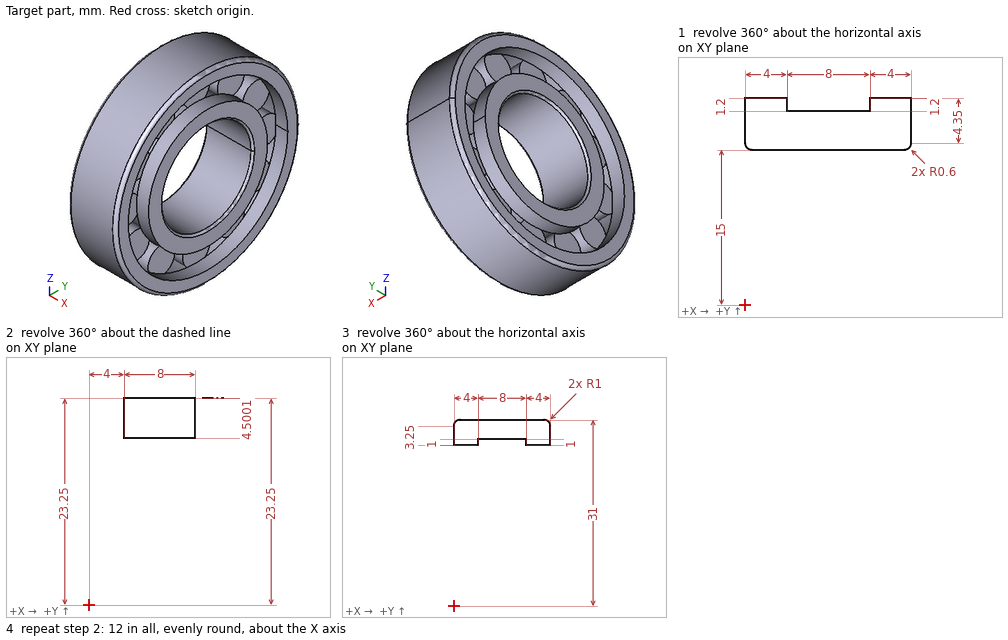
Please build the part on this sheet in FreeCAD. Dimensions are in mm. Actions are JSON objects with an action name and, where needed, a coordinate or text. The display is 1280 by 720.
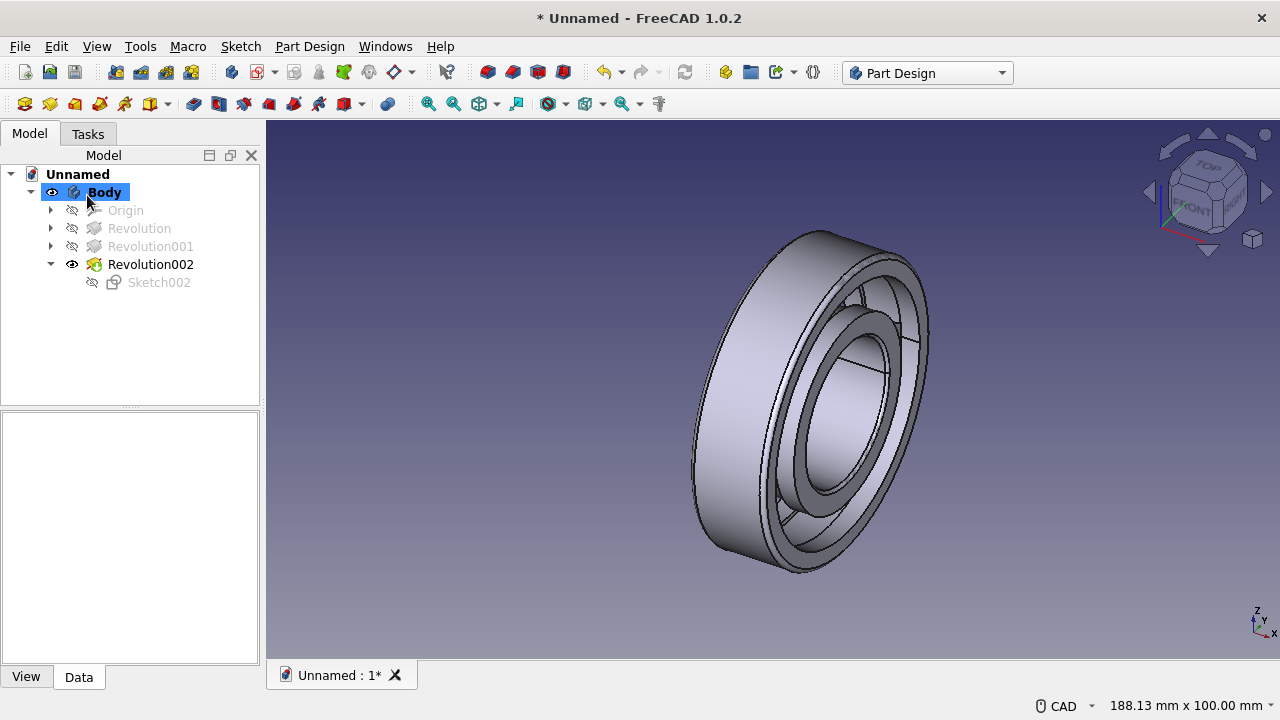
{"action": "left_click", "coordinate": [117, 246]}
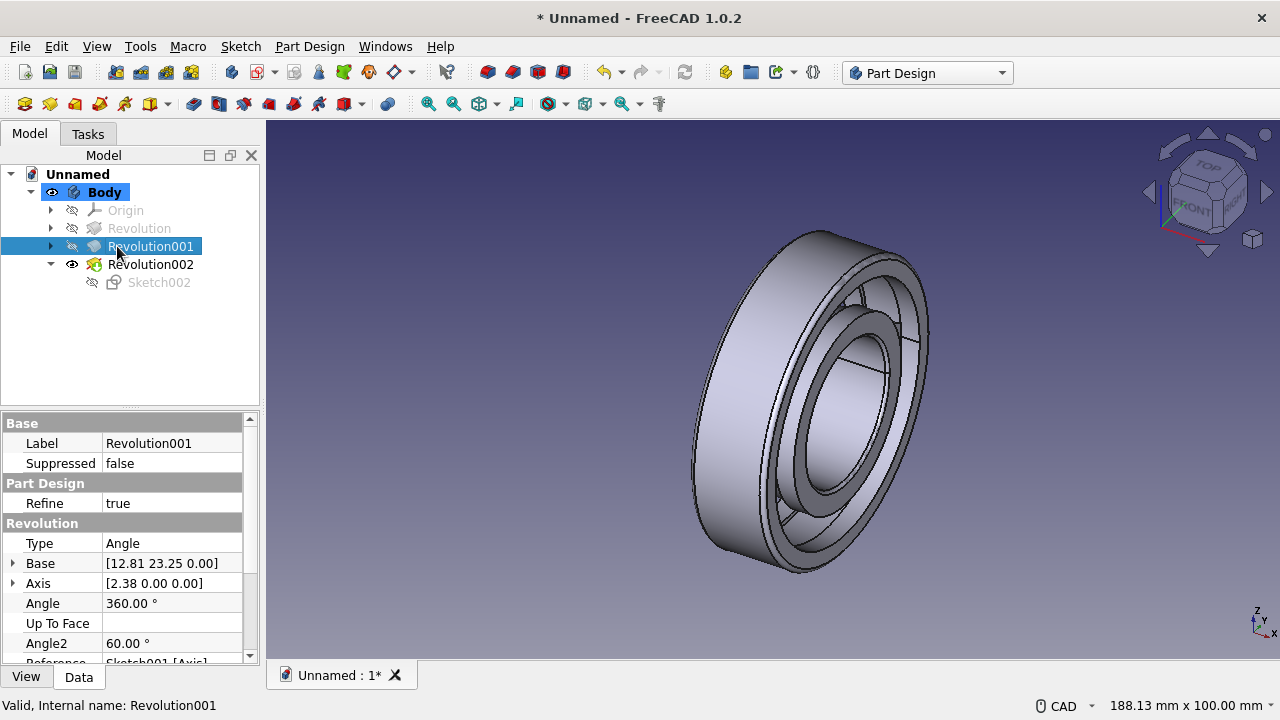
{"action": "left_click", "coordinate": [166, 72]}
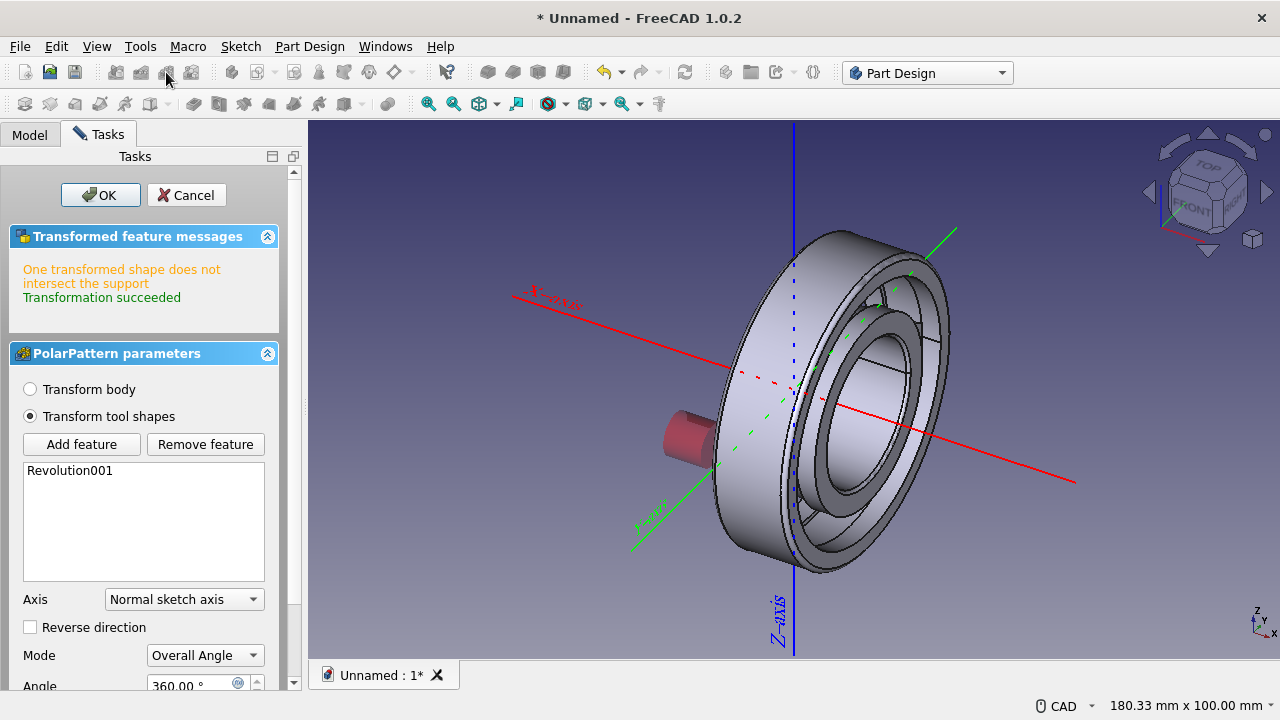
{"action": "left_click", "coordinate": [185, 600]}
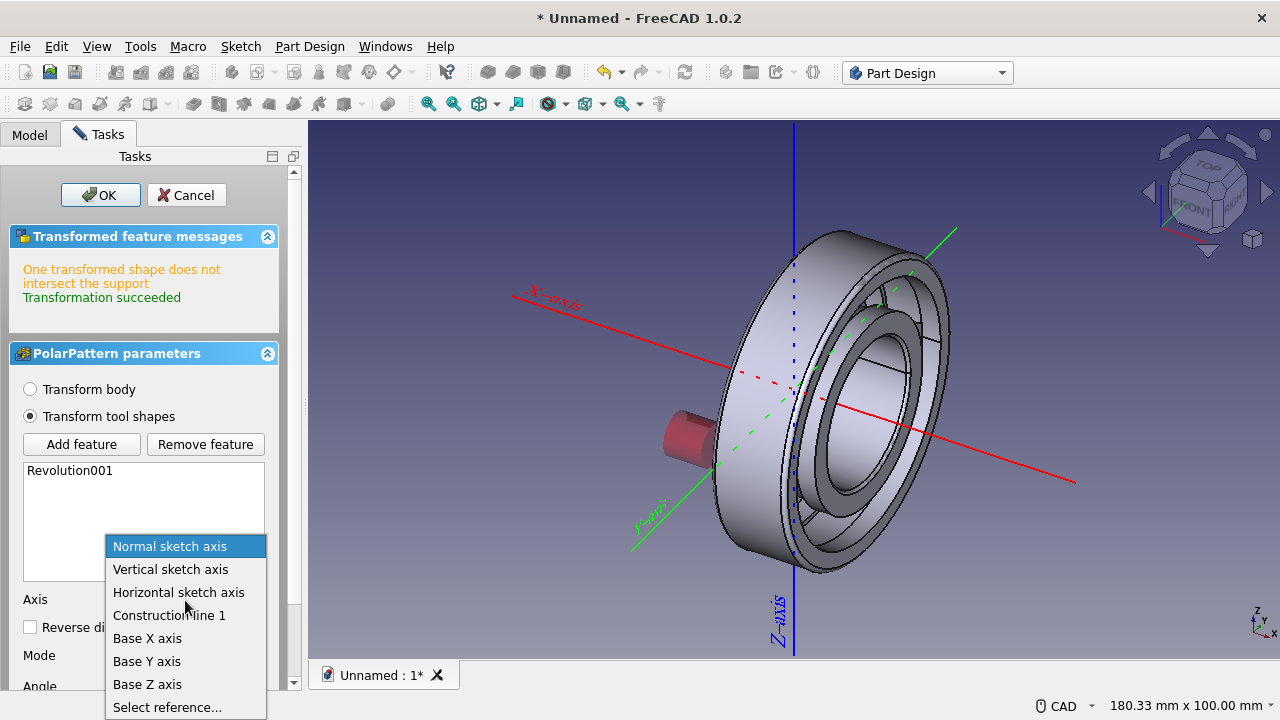
{"action": "left_click", "coordinate": [184, 638]}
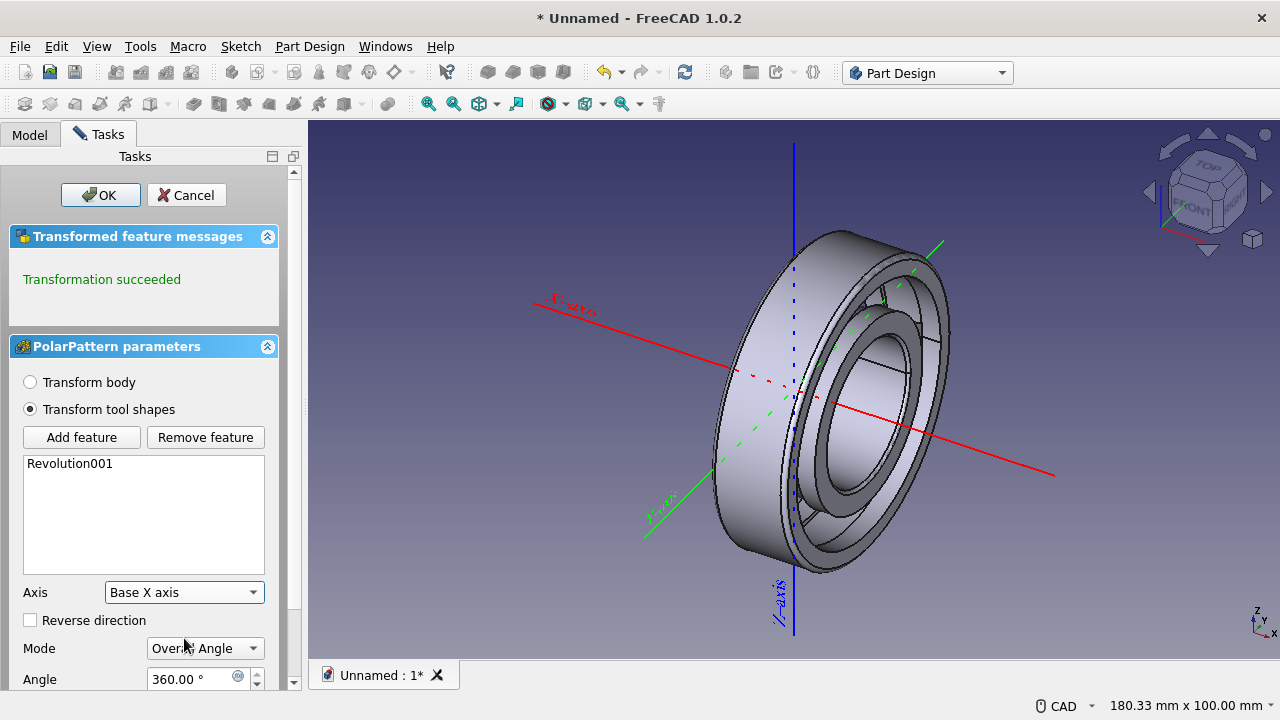
{"action": "scroll", "coordinate": [294, 428], "scroll_direction": "down", "scroll_amount": 2}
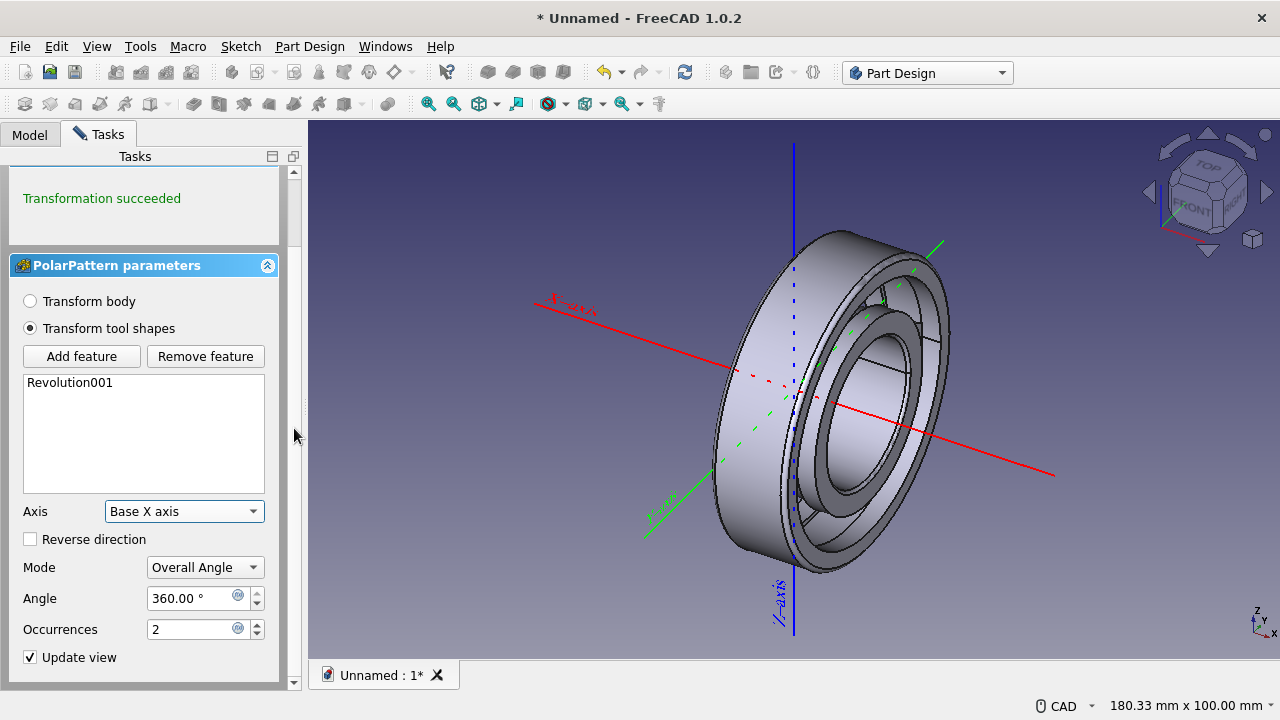
{"action": "triple_click", "coordinate": [199, 630]}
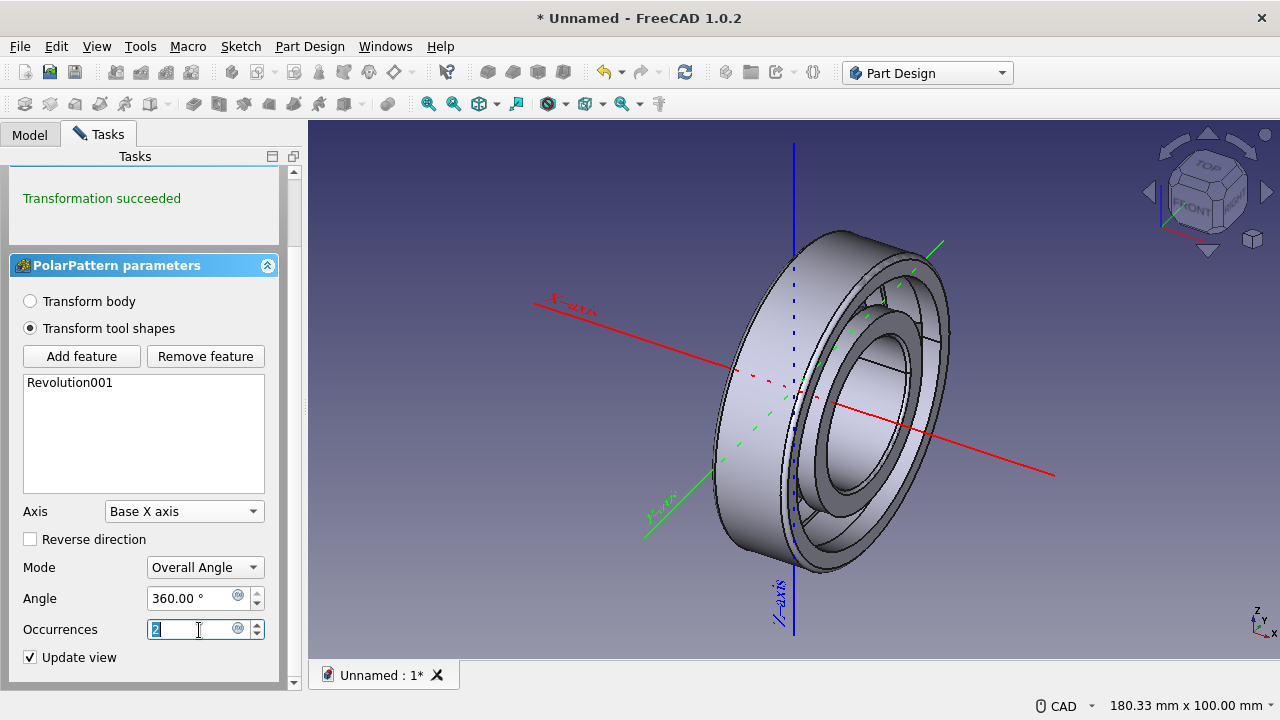
{"action": "type", "text": "12"}
{"action": "key", "text": "Tab"}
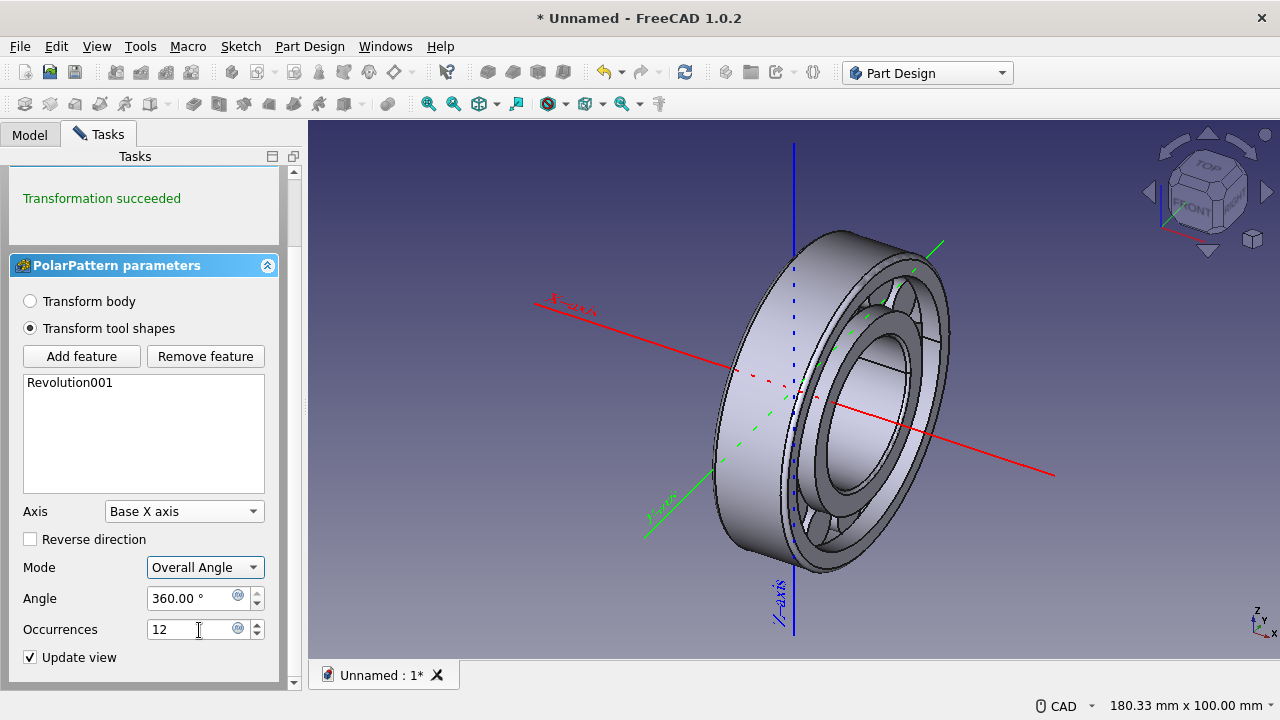
{"action": "scroll", "coordinate": [294, 428], "scroll_direction": "up", "scroll_amount": 3}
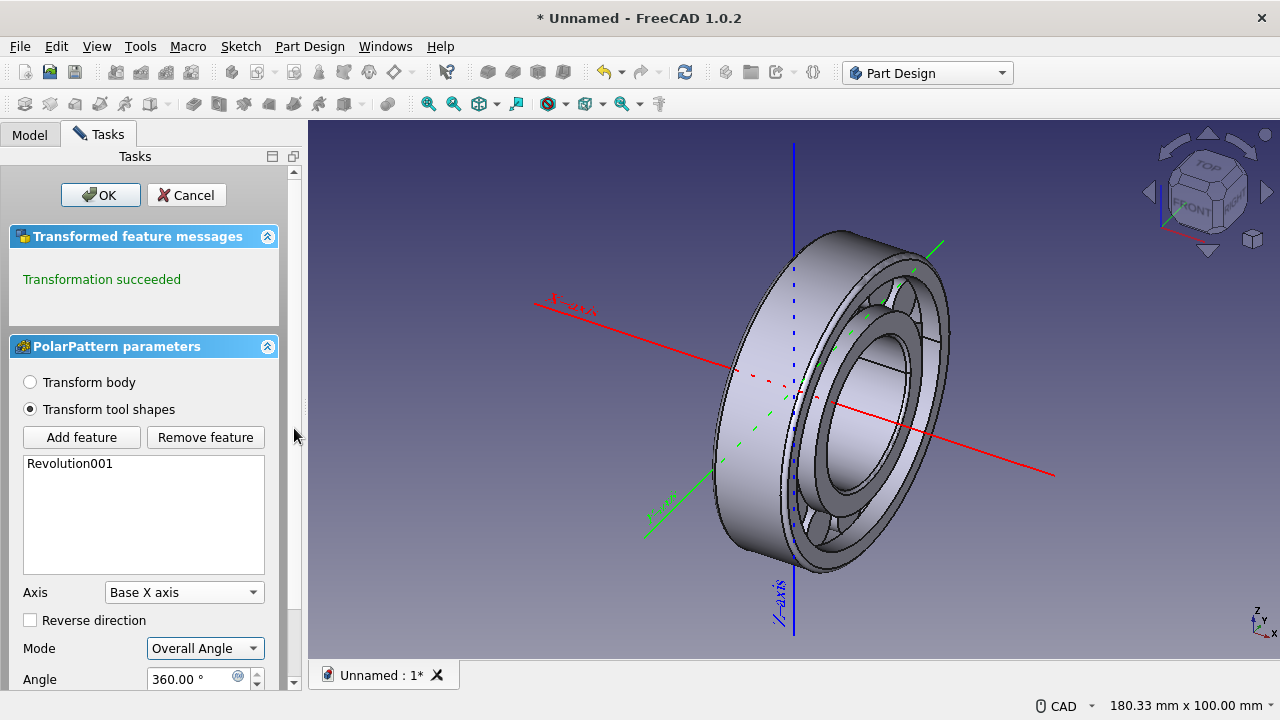
{"action": "left_click", "coordinate": [101, 195]}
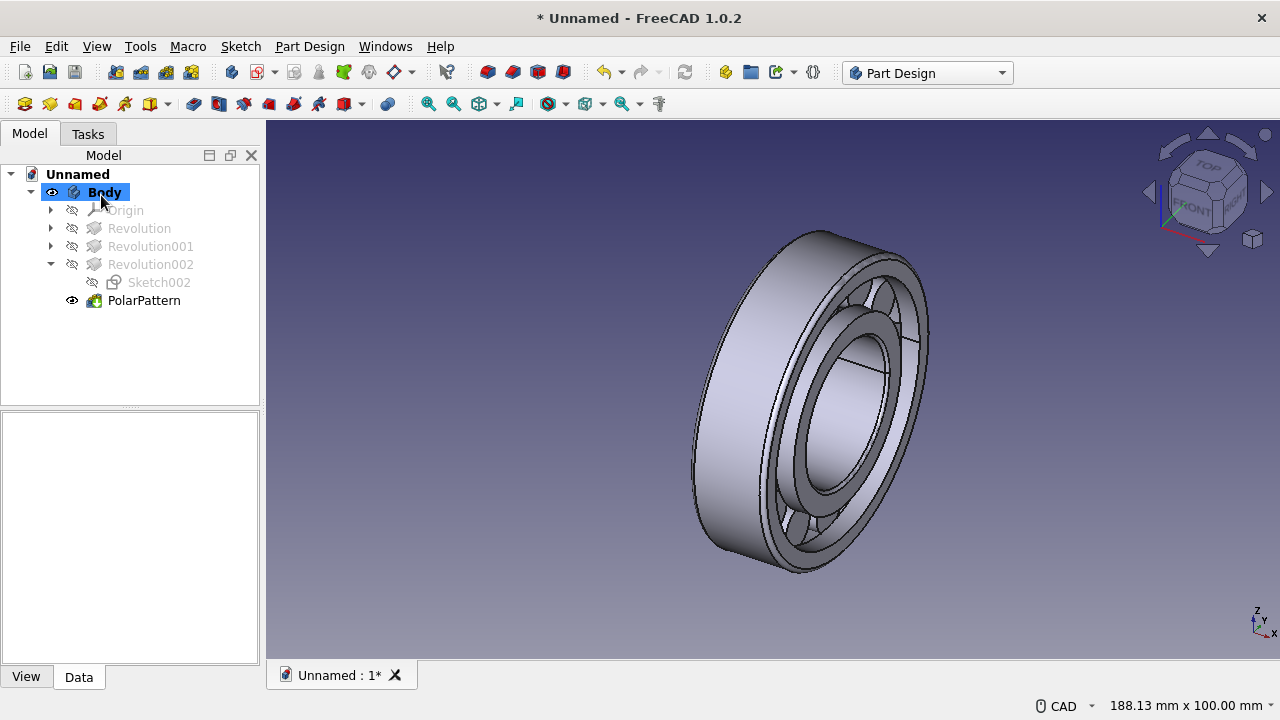
{"action": "key", "text": "0"}